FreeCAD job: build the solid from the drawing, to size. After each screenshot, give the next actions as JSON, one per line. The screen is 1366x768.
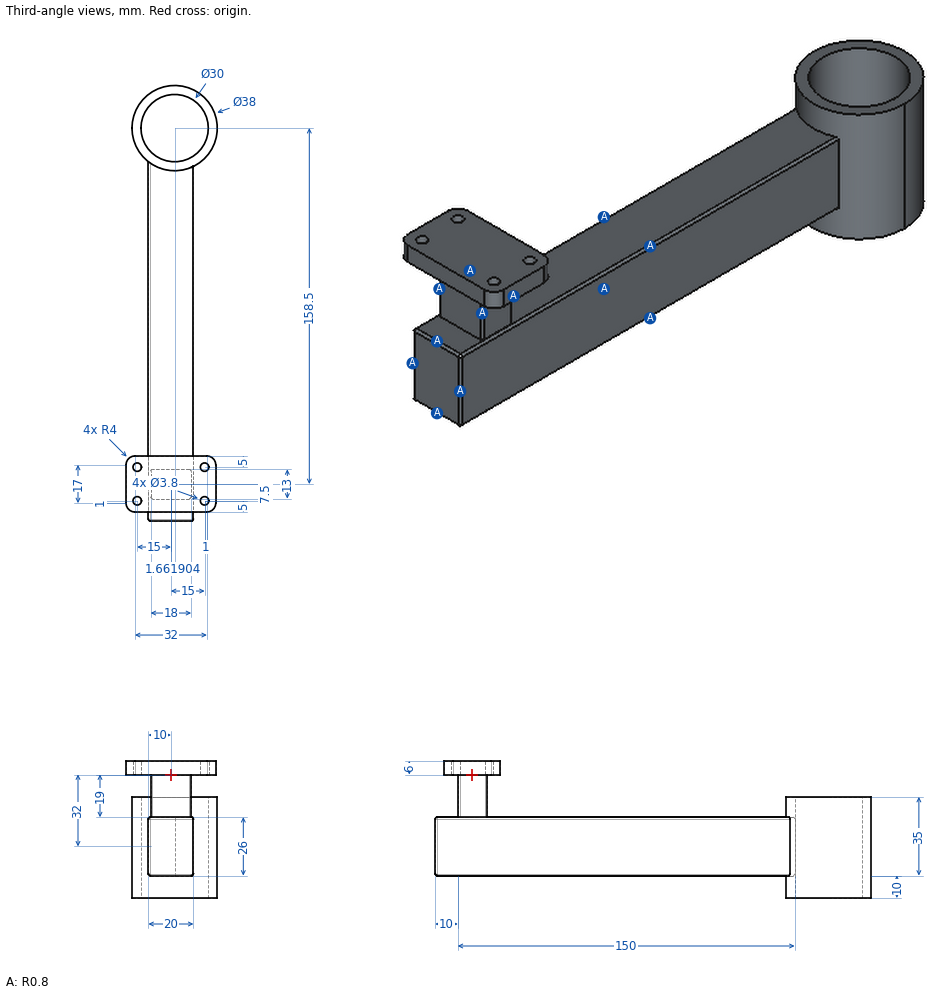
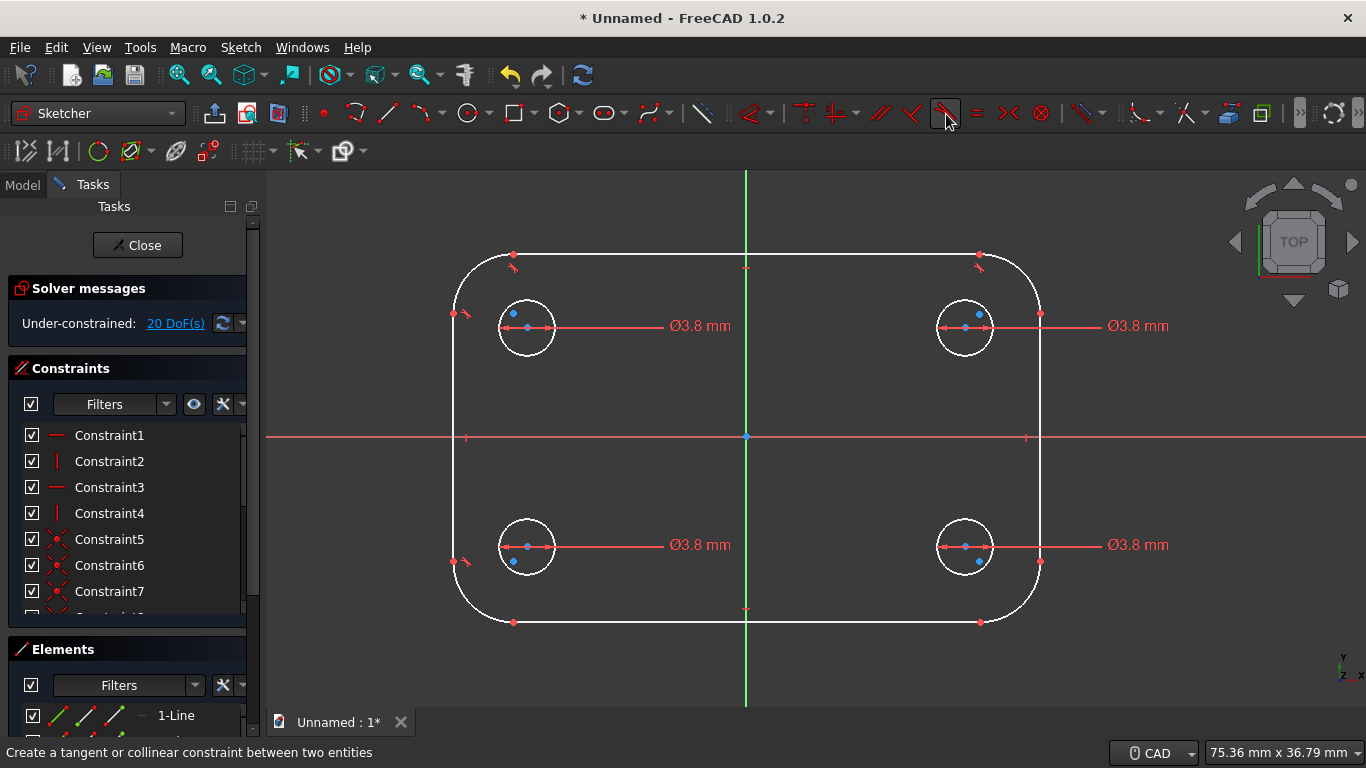
{"action": "left_click", "coordinate": [653, 622]}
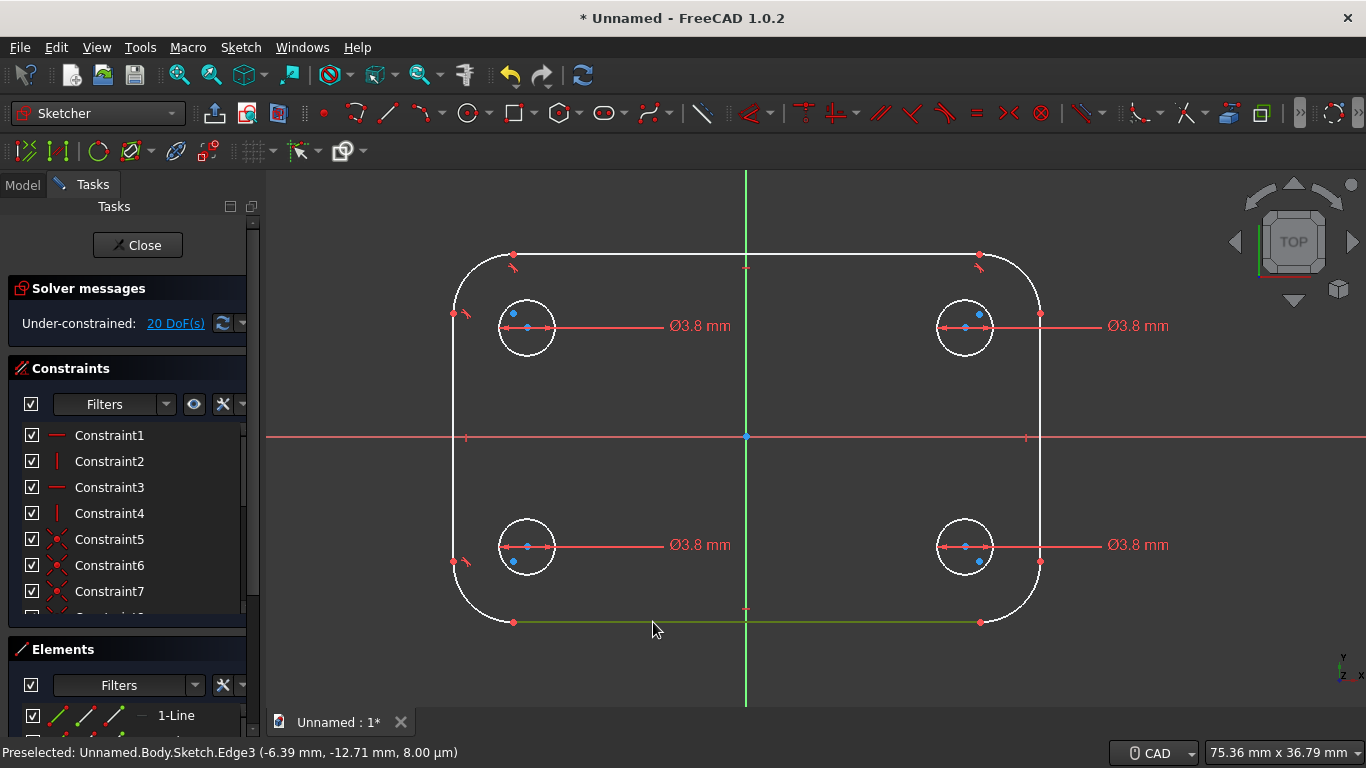
{"action": "left_click", "coordinate": [460, 589]}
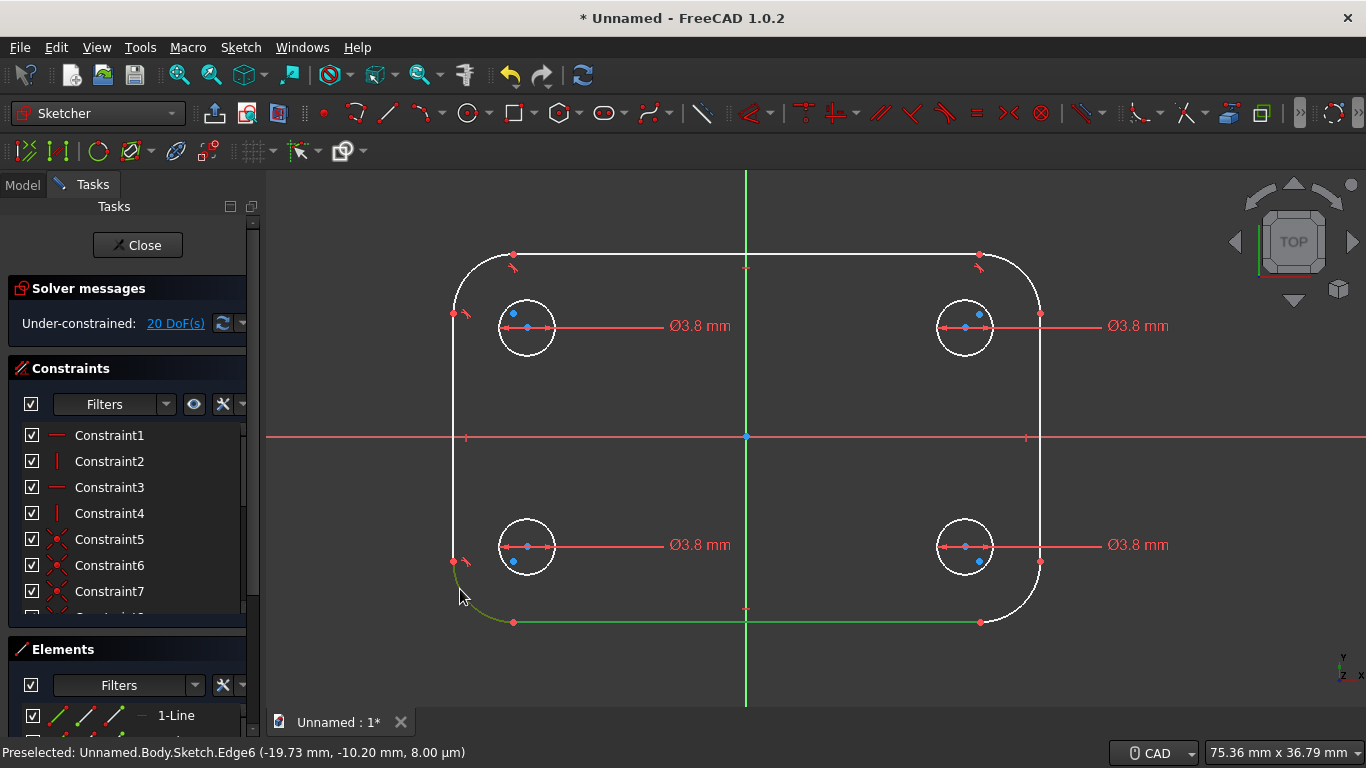
{"action": "key", "text": "t"}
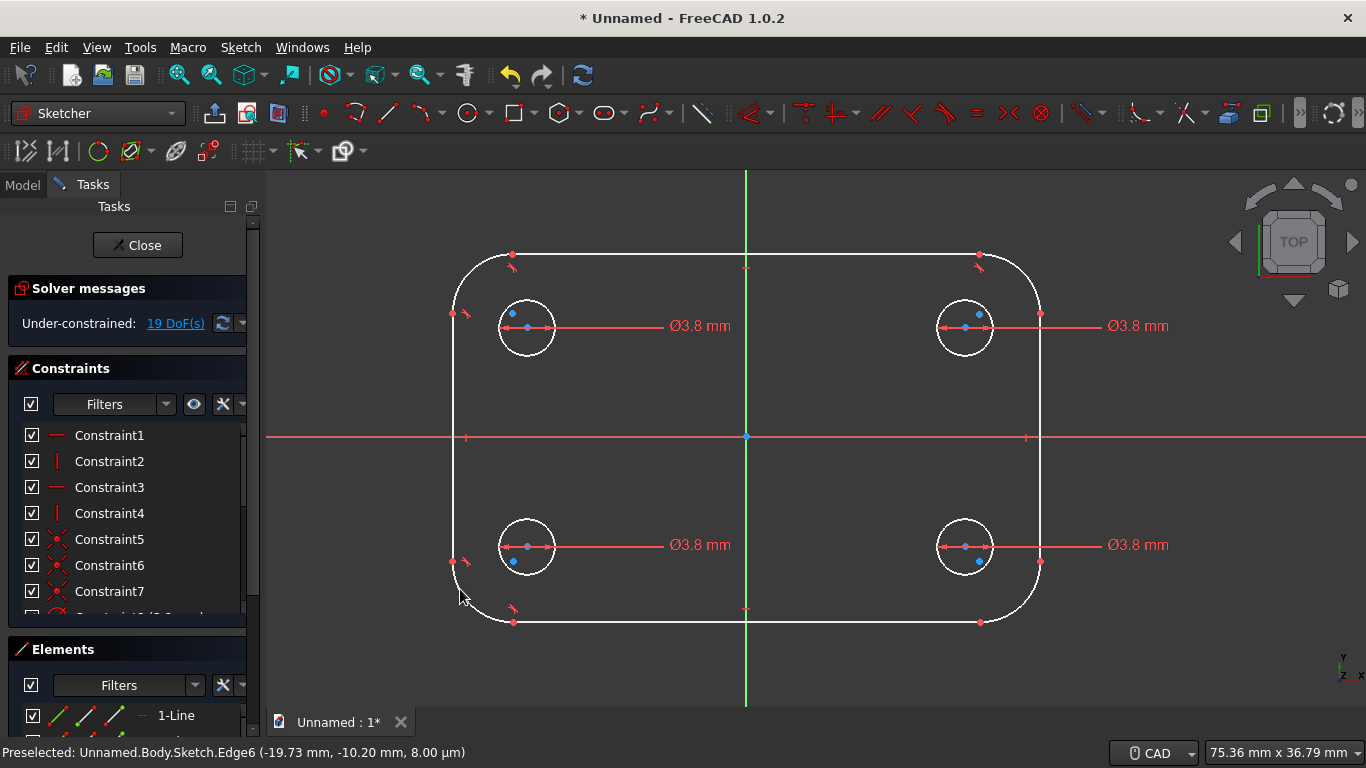
{"action": "left_click", "coordinate": [653, 622]}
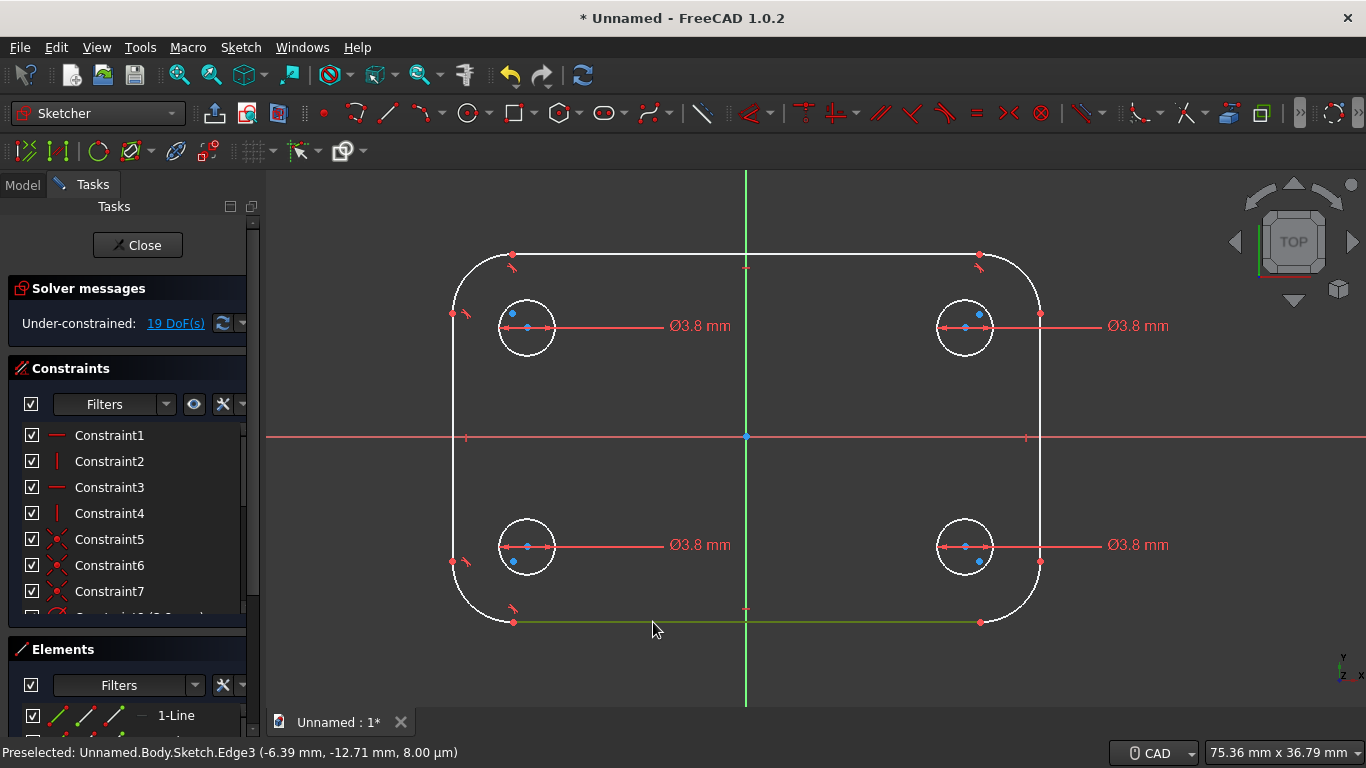
{"action": "left_click", "coordinate": [1007, 616]}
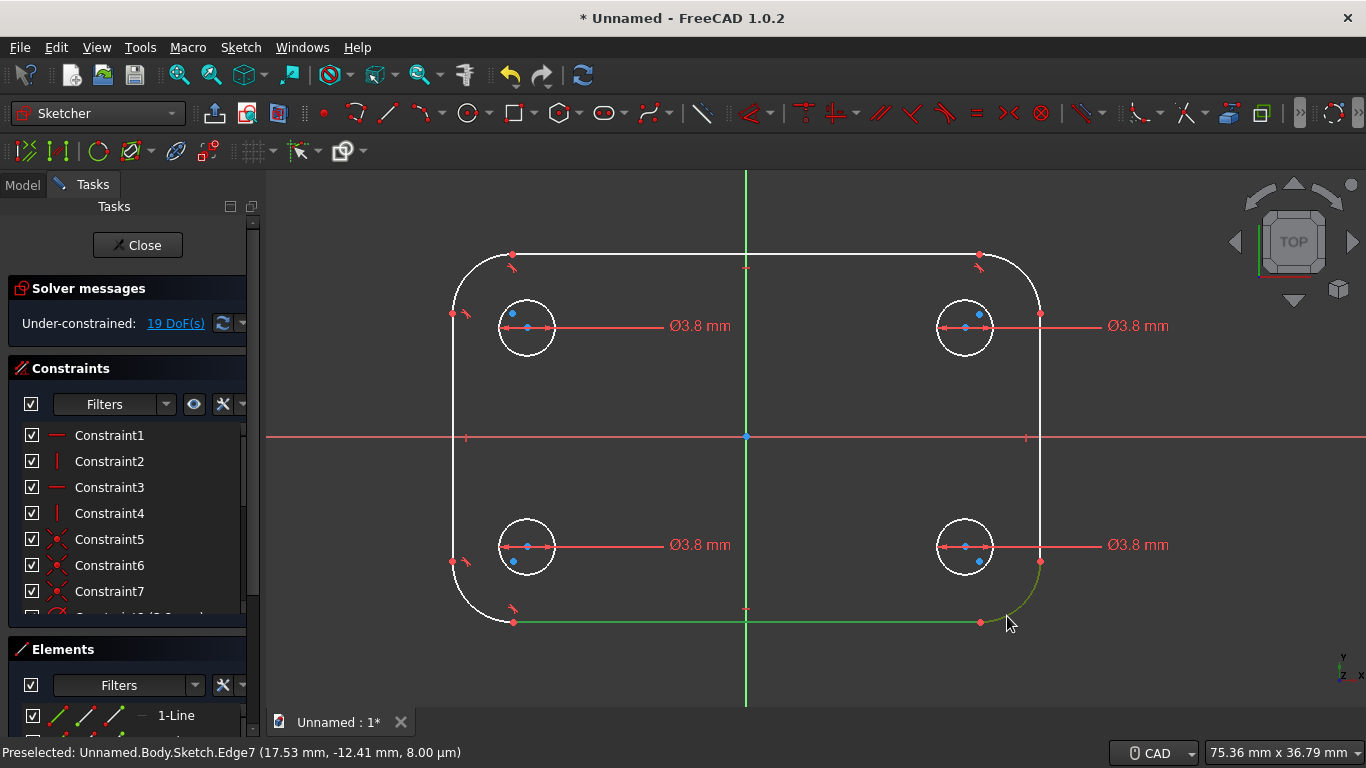
{"action": "left_click", "coordinate": [946, 114]}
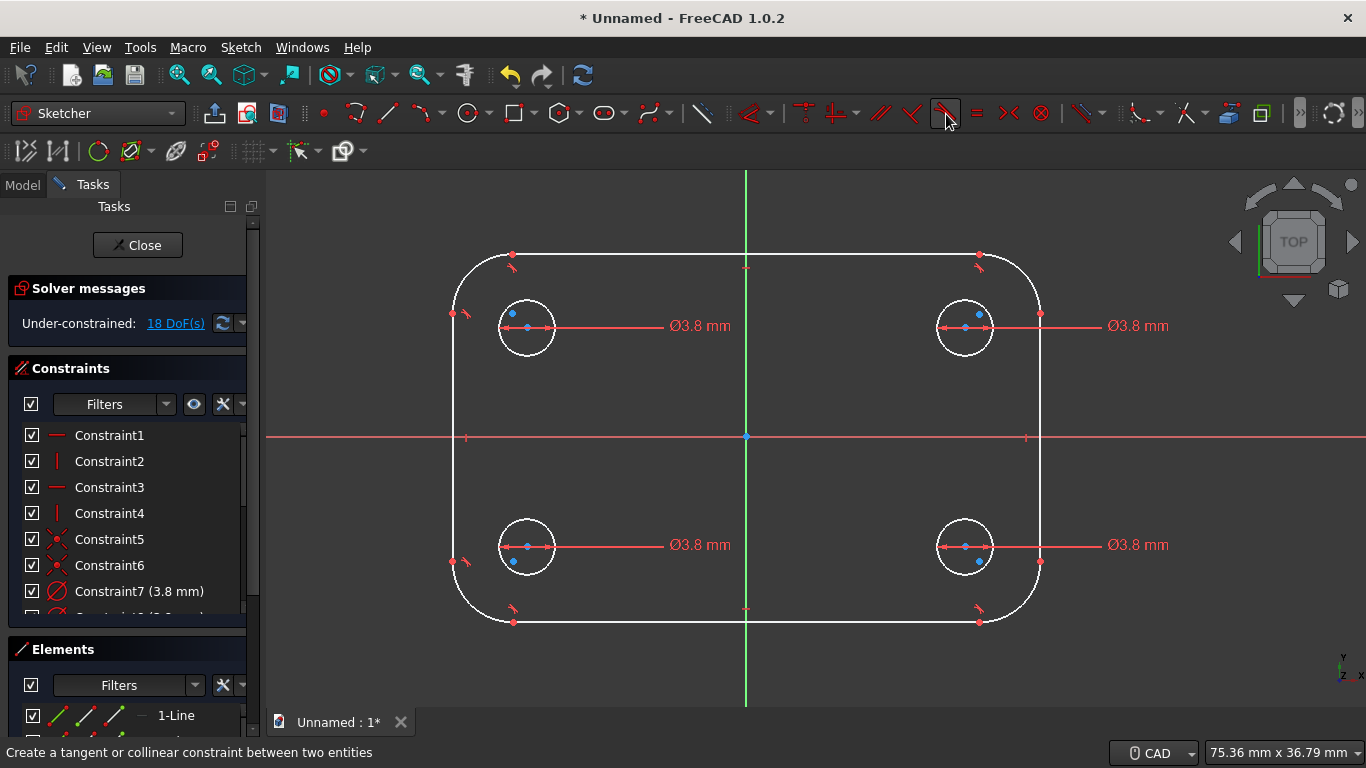
{"action": "left_click", "coordinate": [1040, 488]}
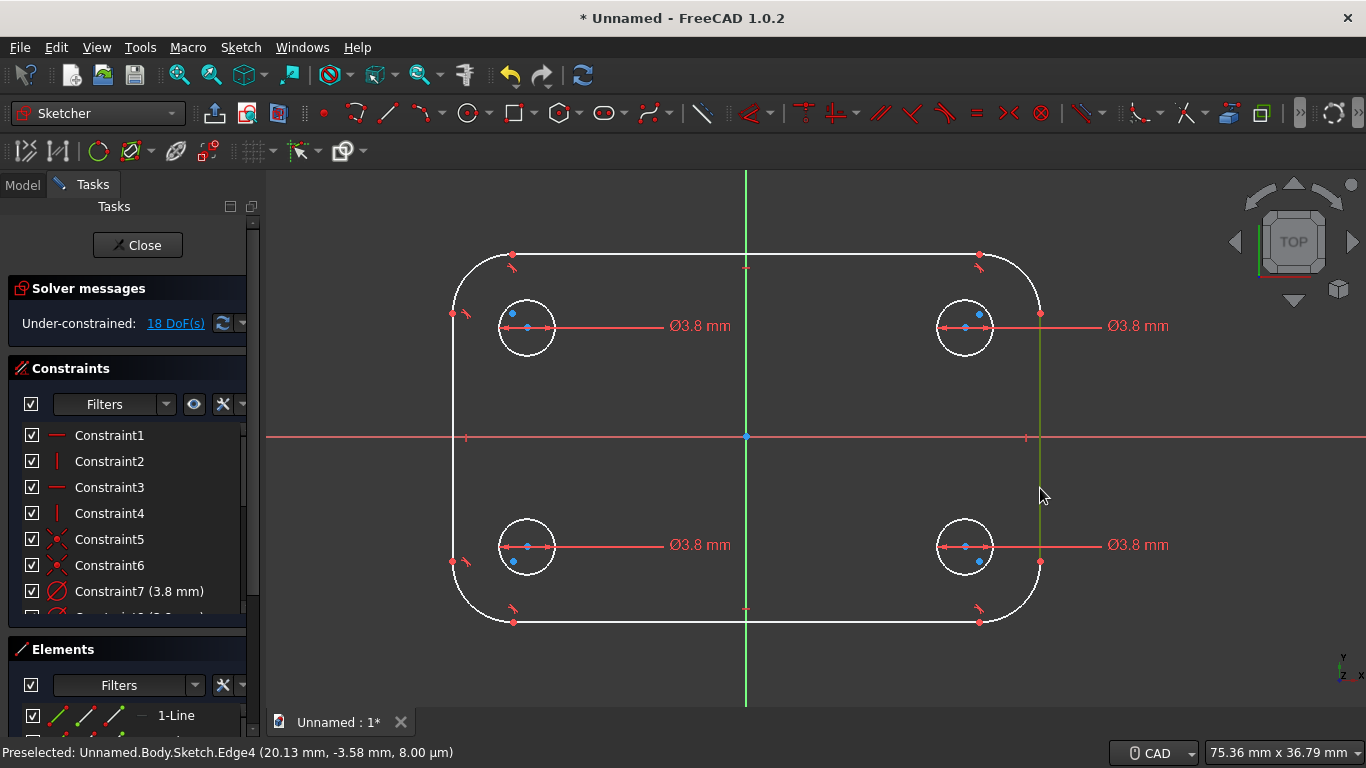
{"action": "left_click", "coordinate": [1007, 616]}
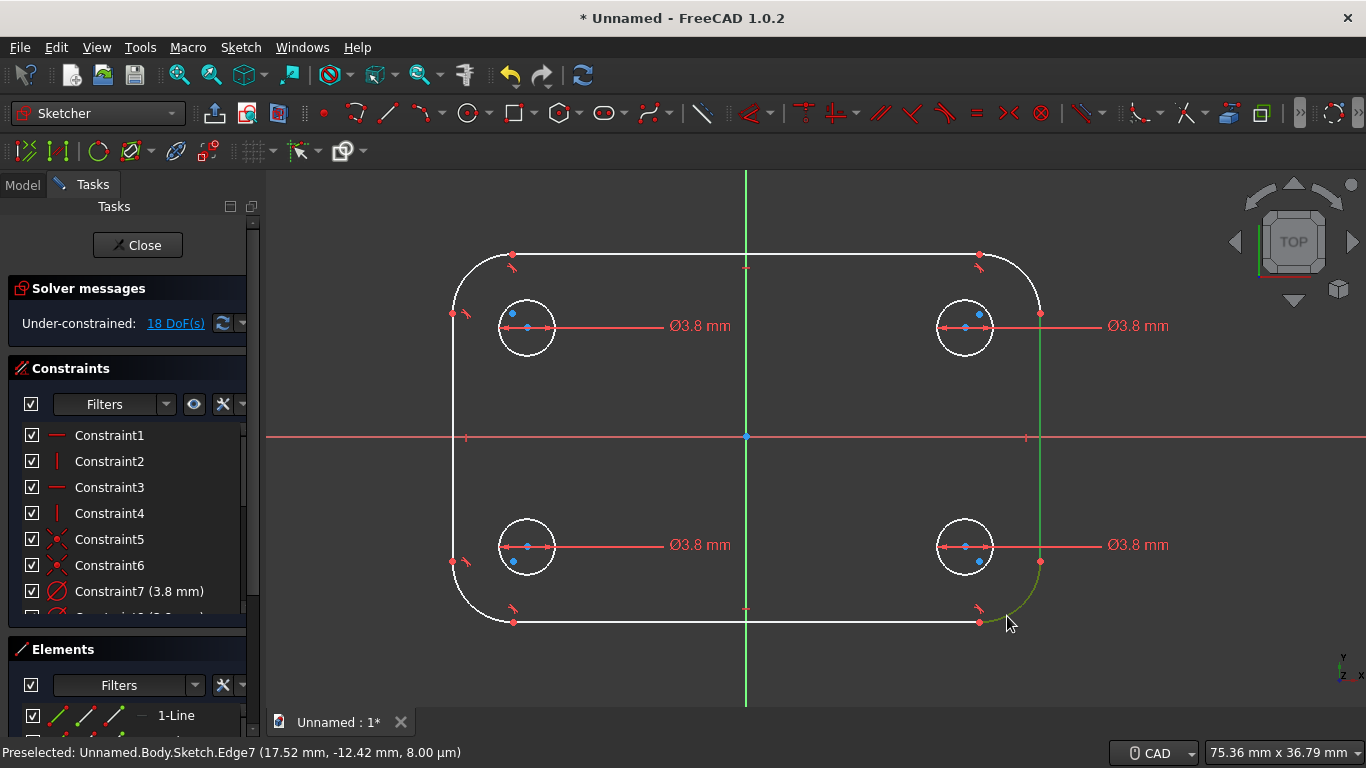
{"action": "key", "text": "t"}